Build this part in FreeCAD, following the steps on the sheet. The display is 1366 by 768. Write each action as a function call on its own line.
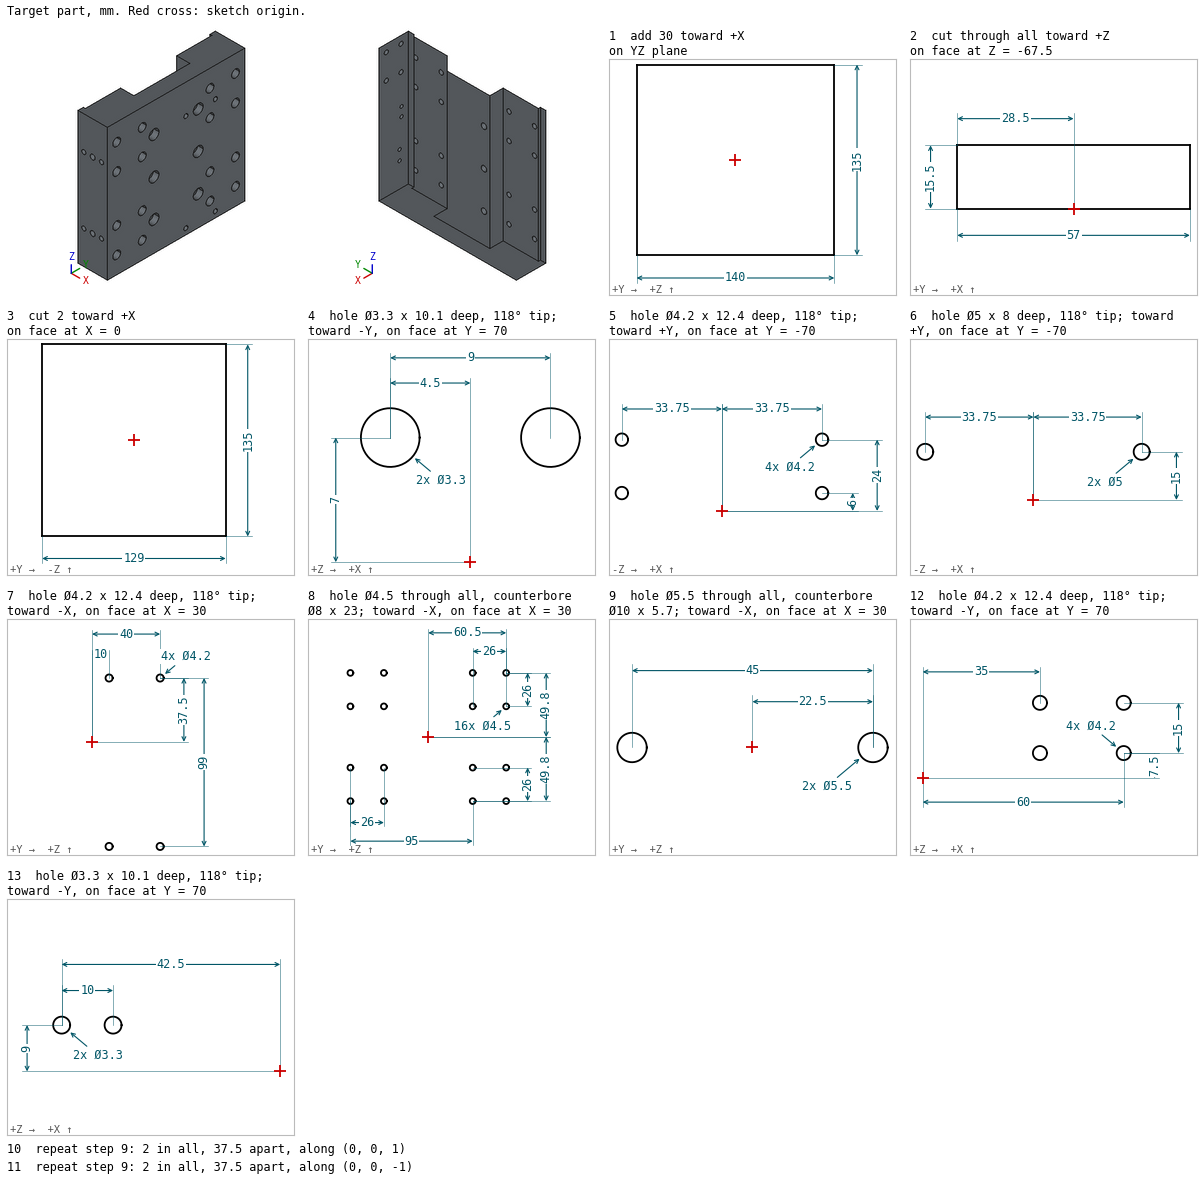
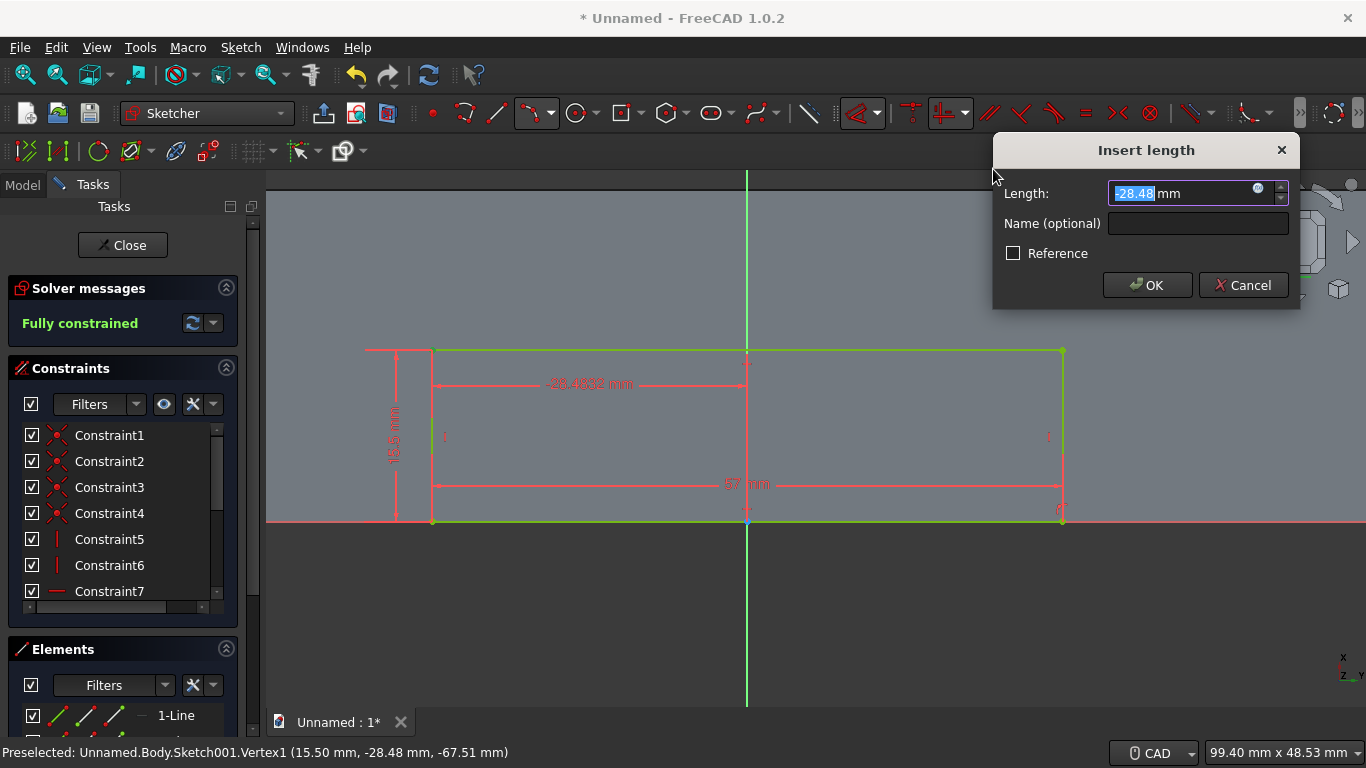
text(-28.5)
key(Return)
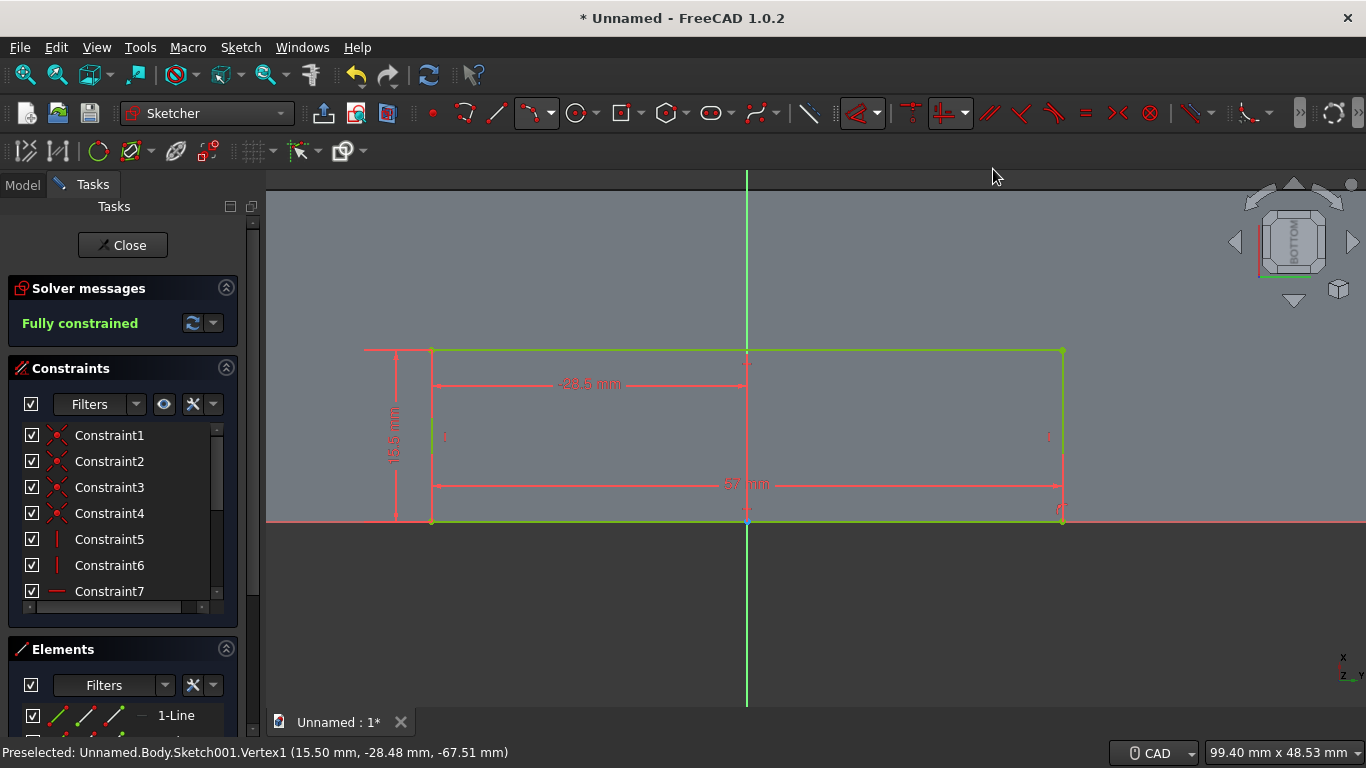
click(123, 245)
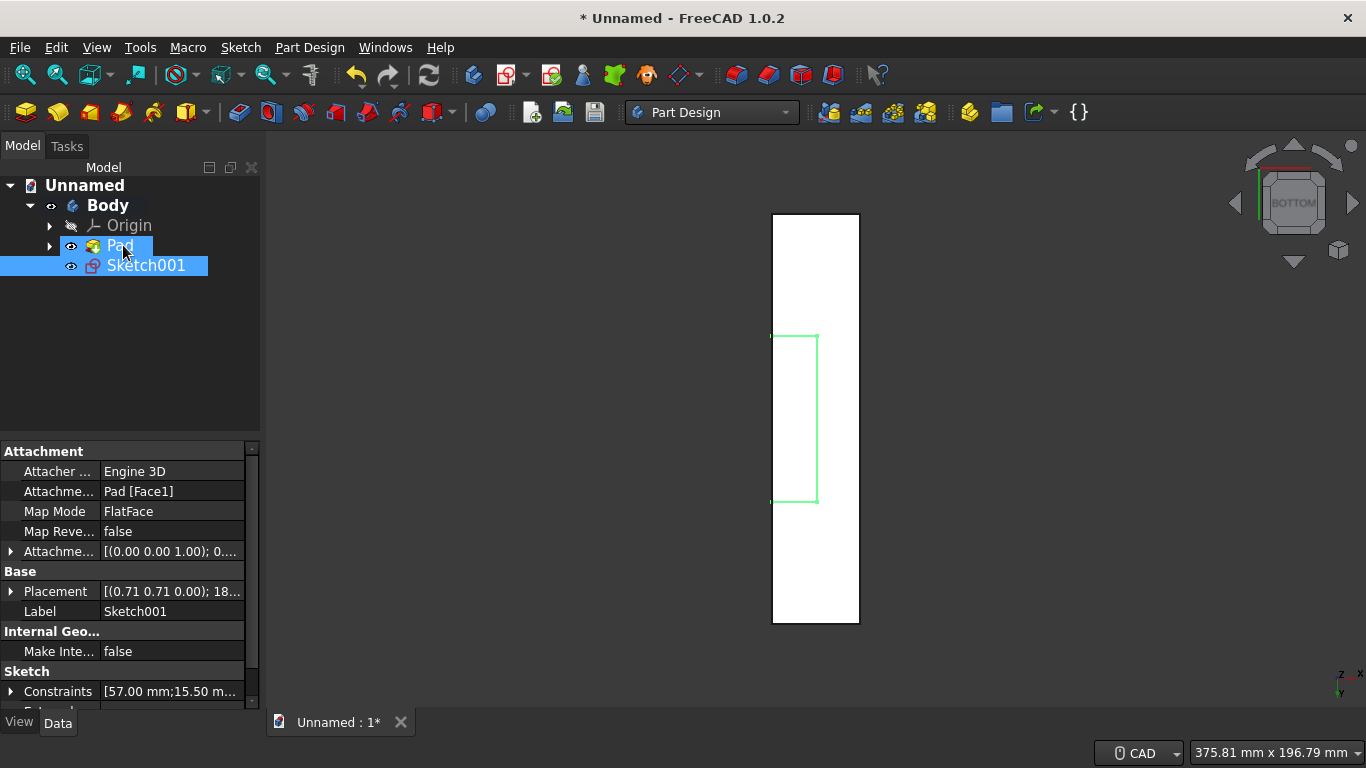
click(240, 112)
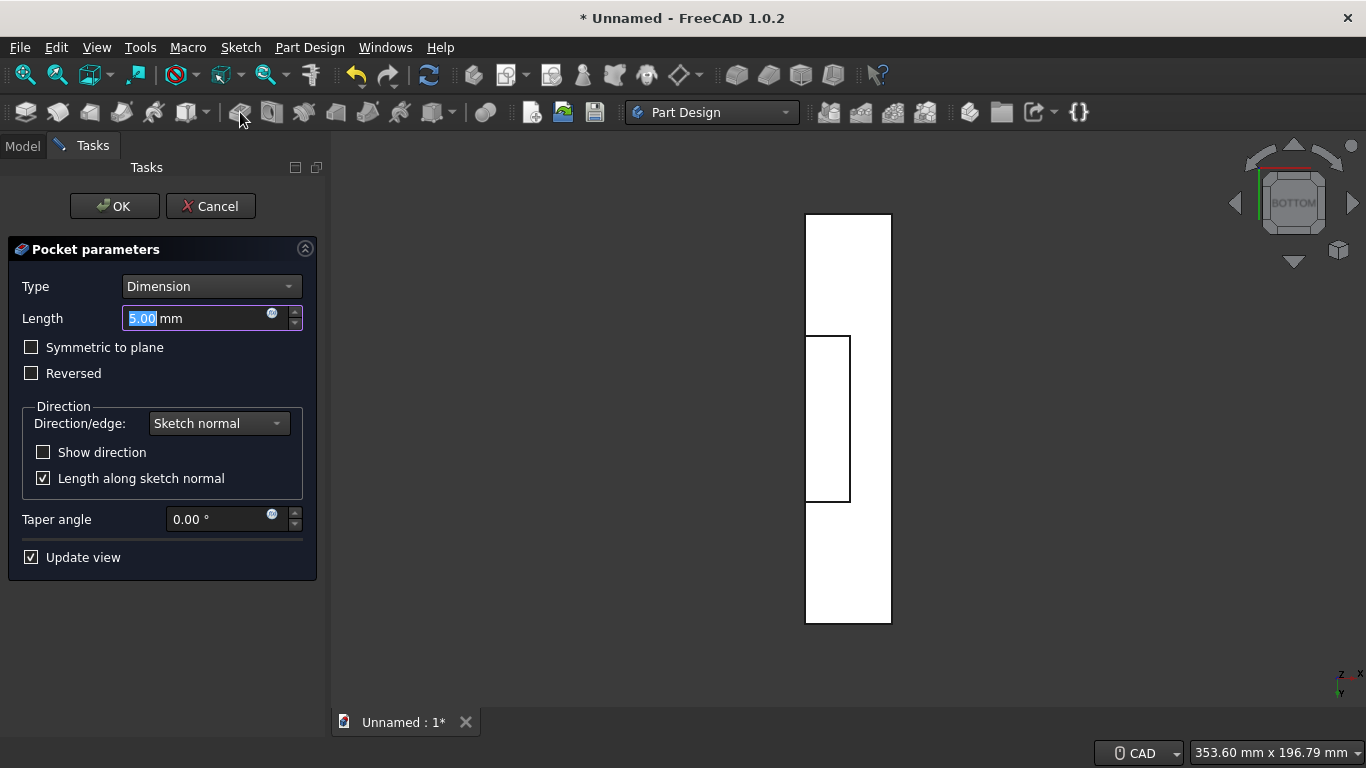
click(212, 286)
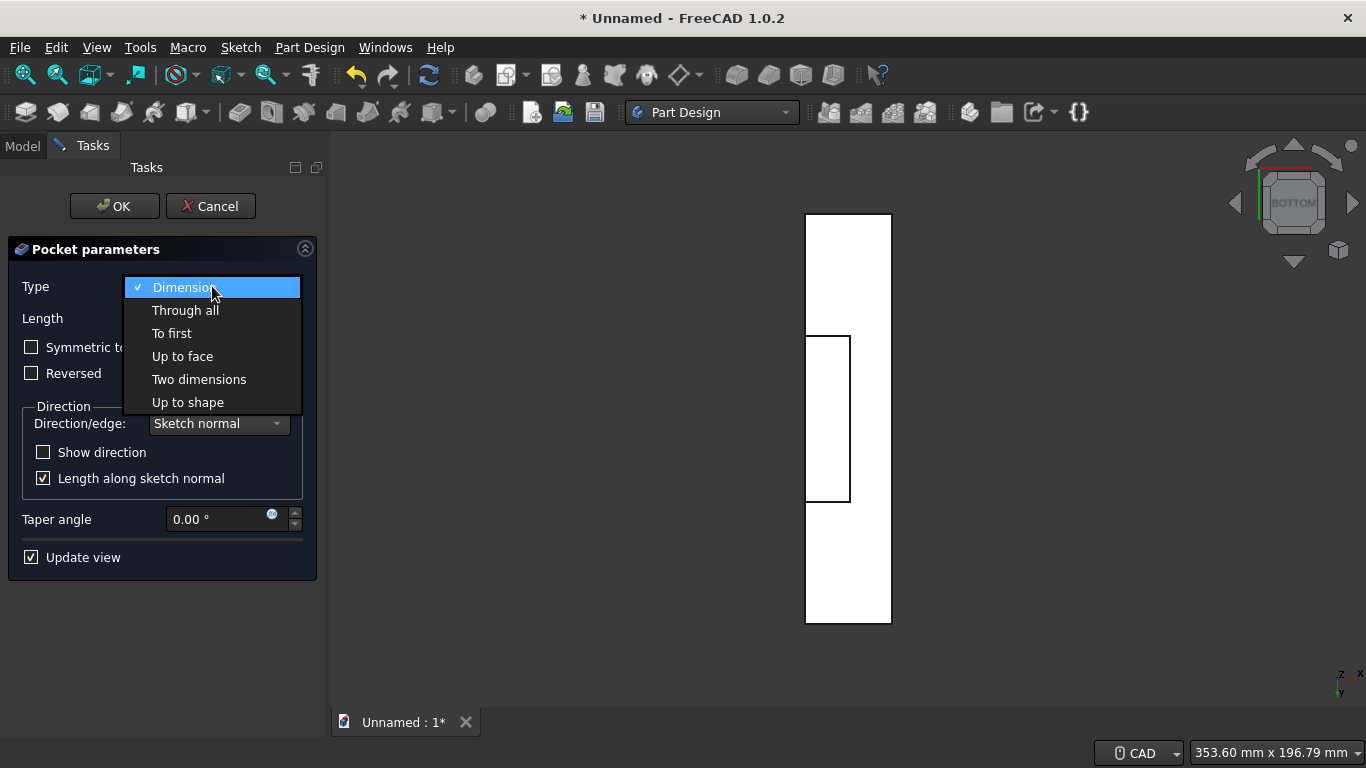
click(212, 310)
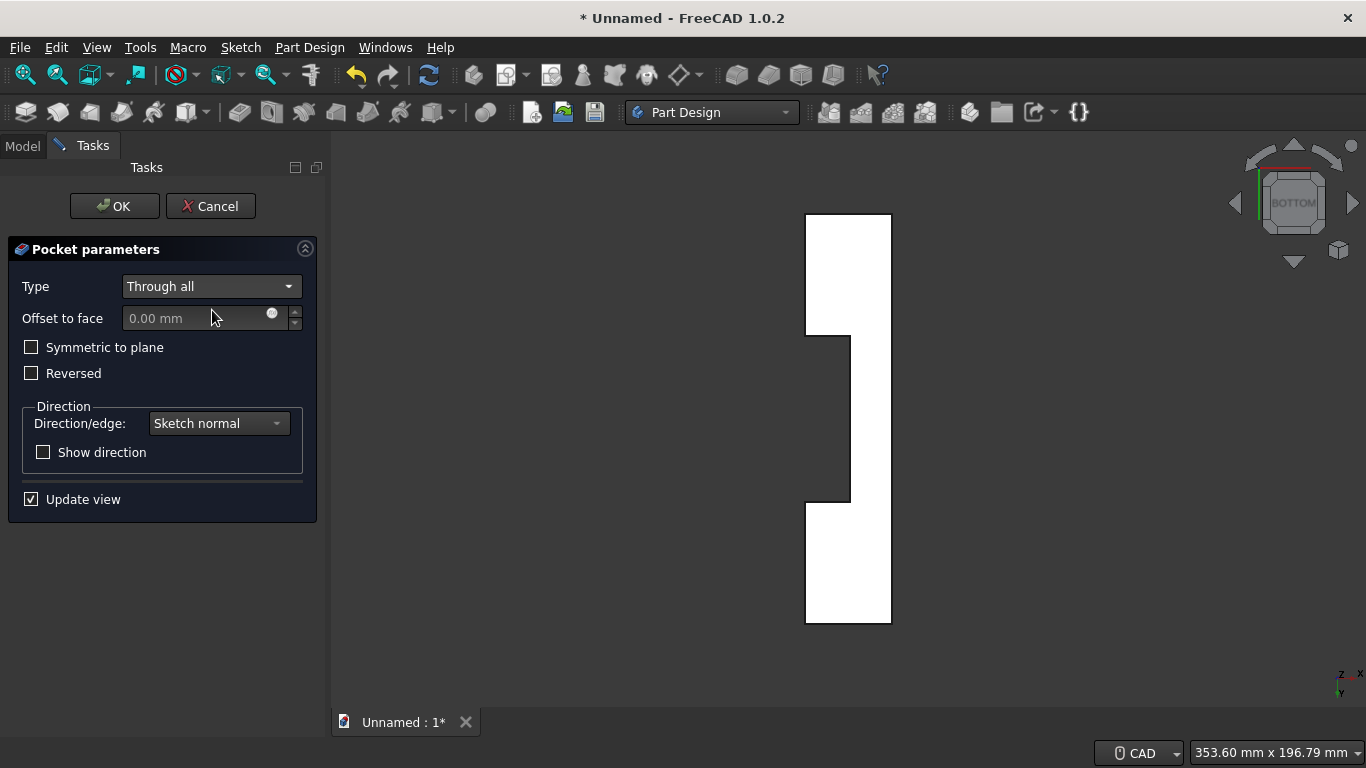
click(115, 206)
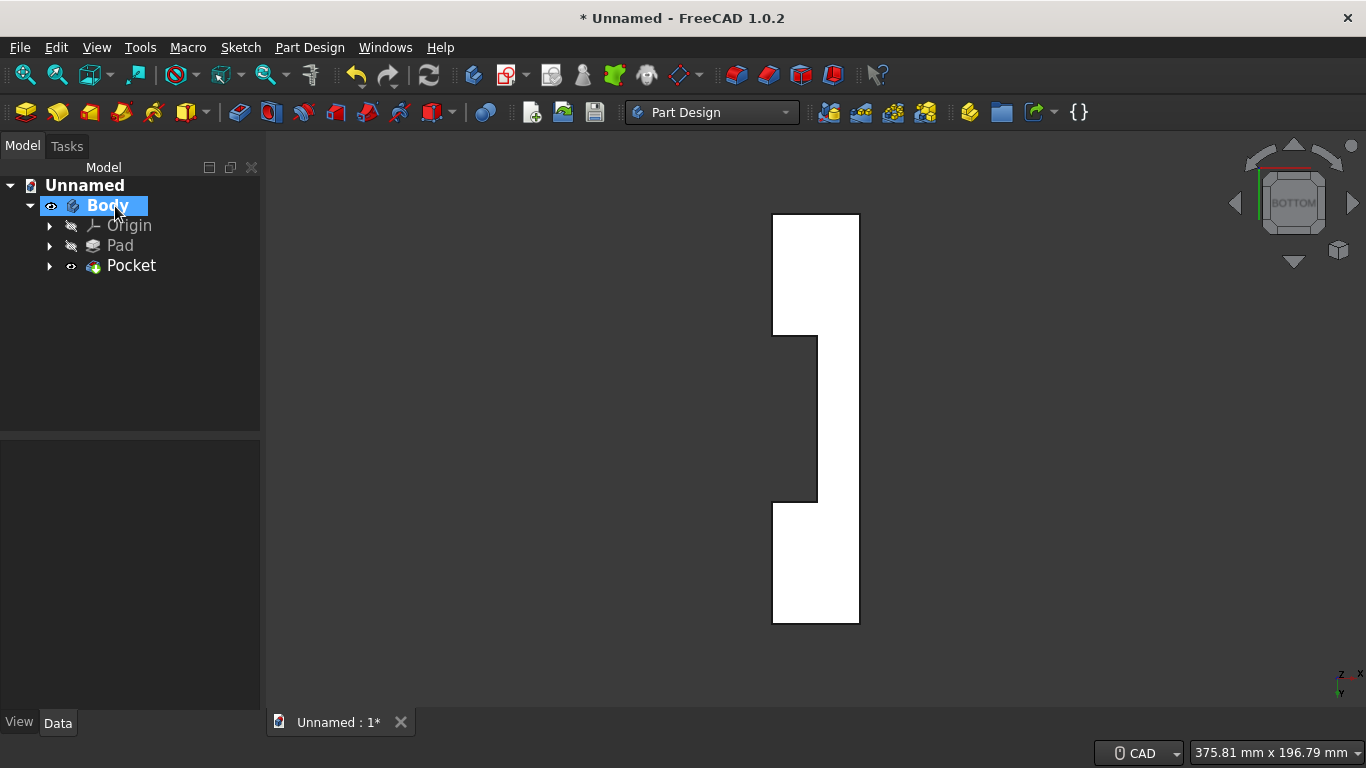
key(6)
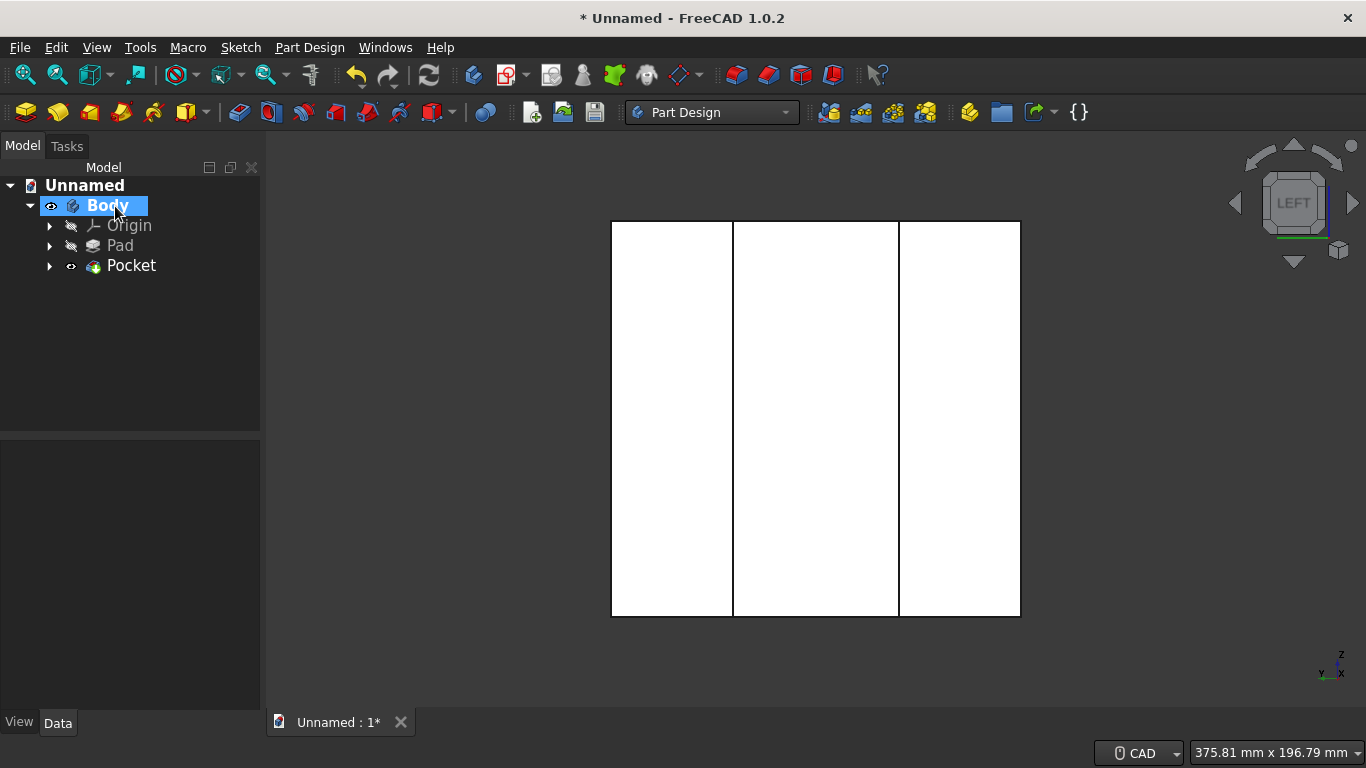
click(672, 362)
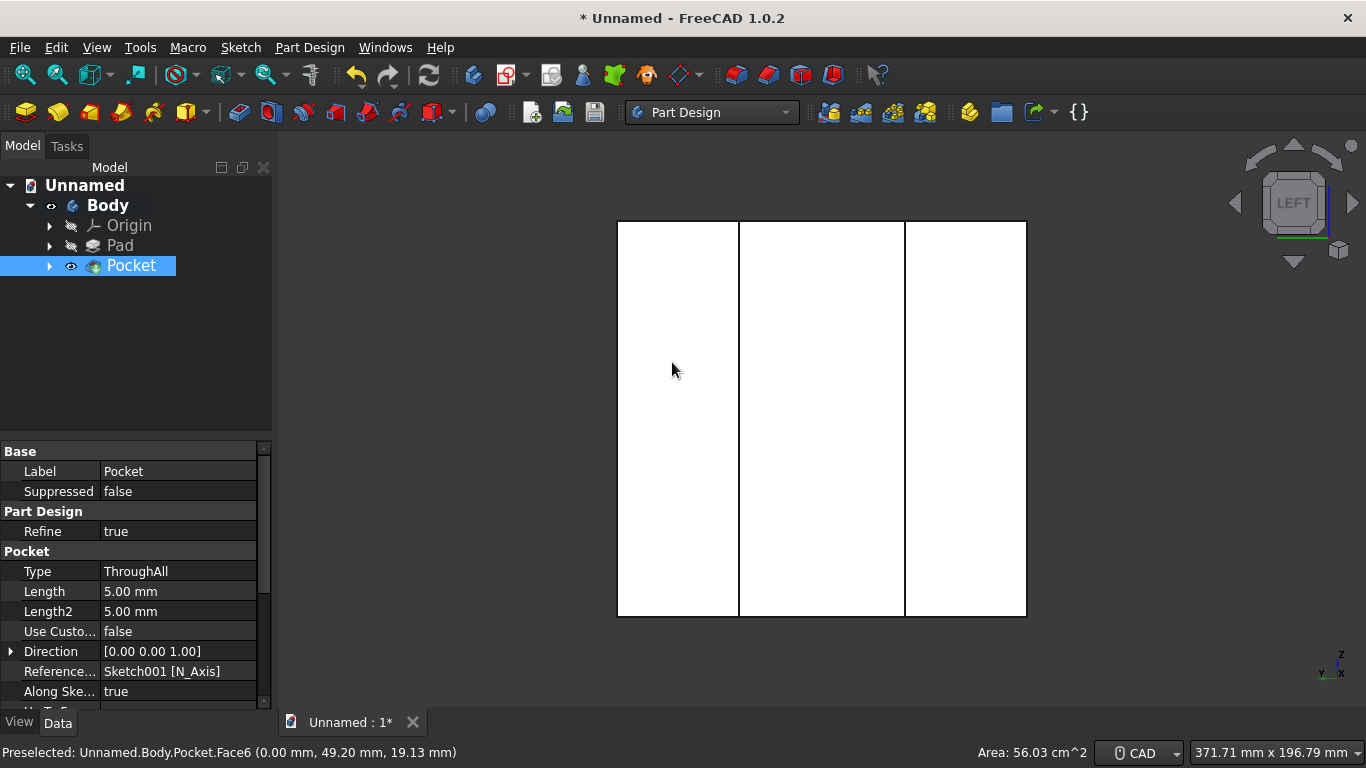
click(506, 76)